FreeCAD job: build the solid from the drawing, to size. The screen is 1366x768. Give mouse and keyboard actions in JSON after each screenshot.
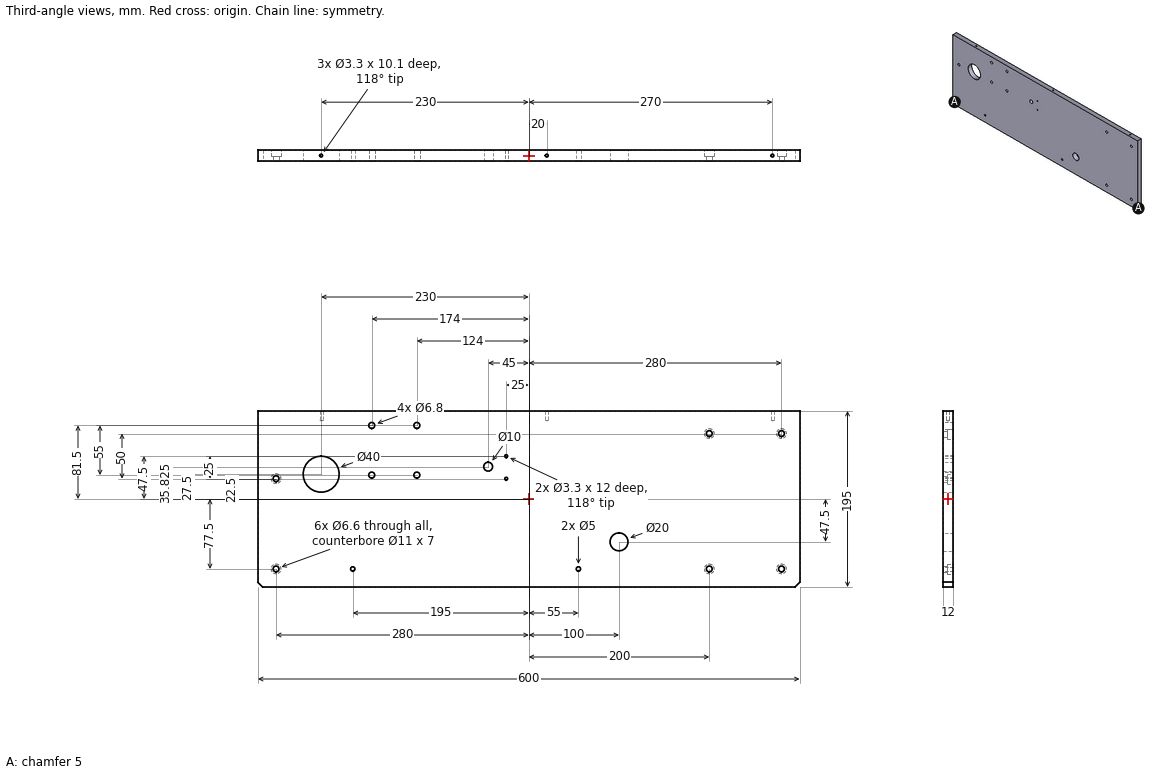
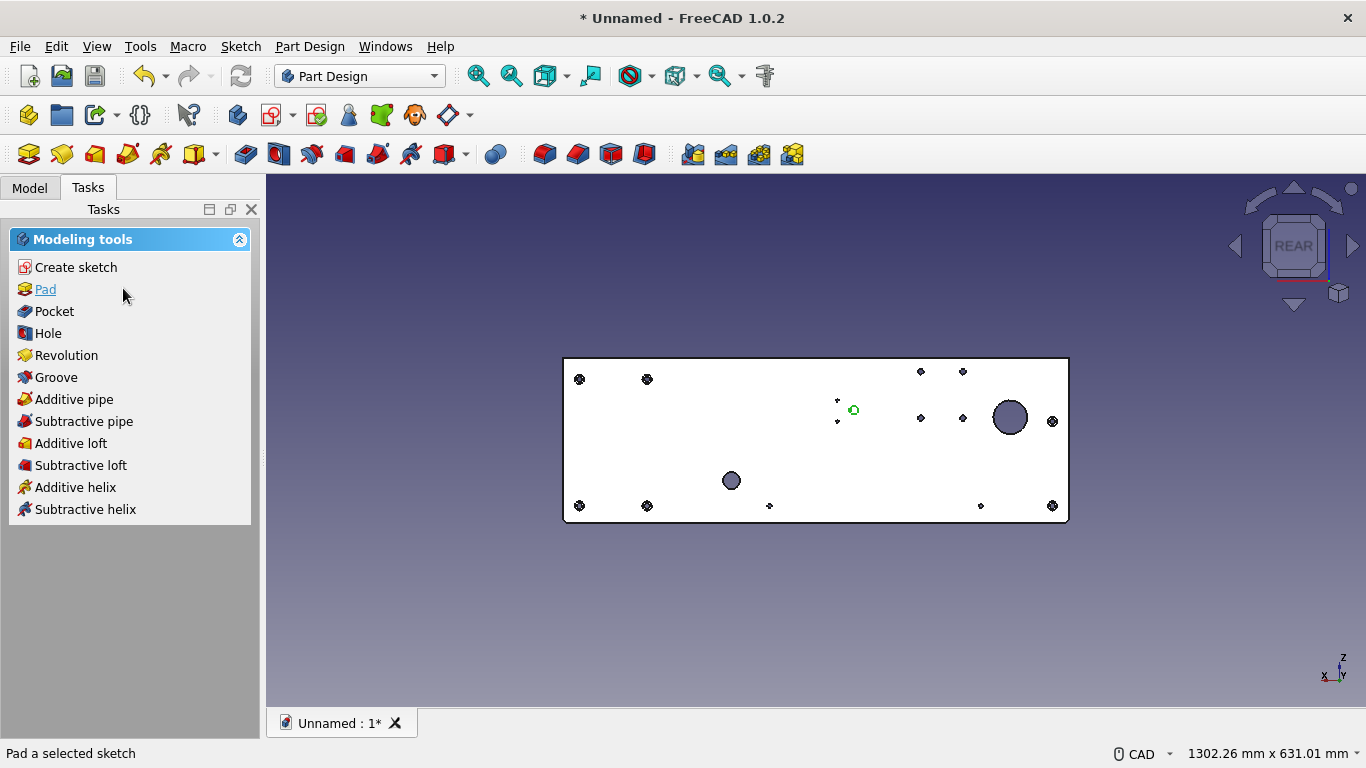
{"action": "left_click", "coordinate": [246, 154]}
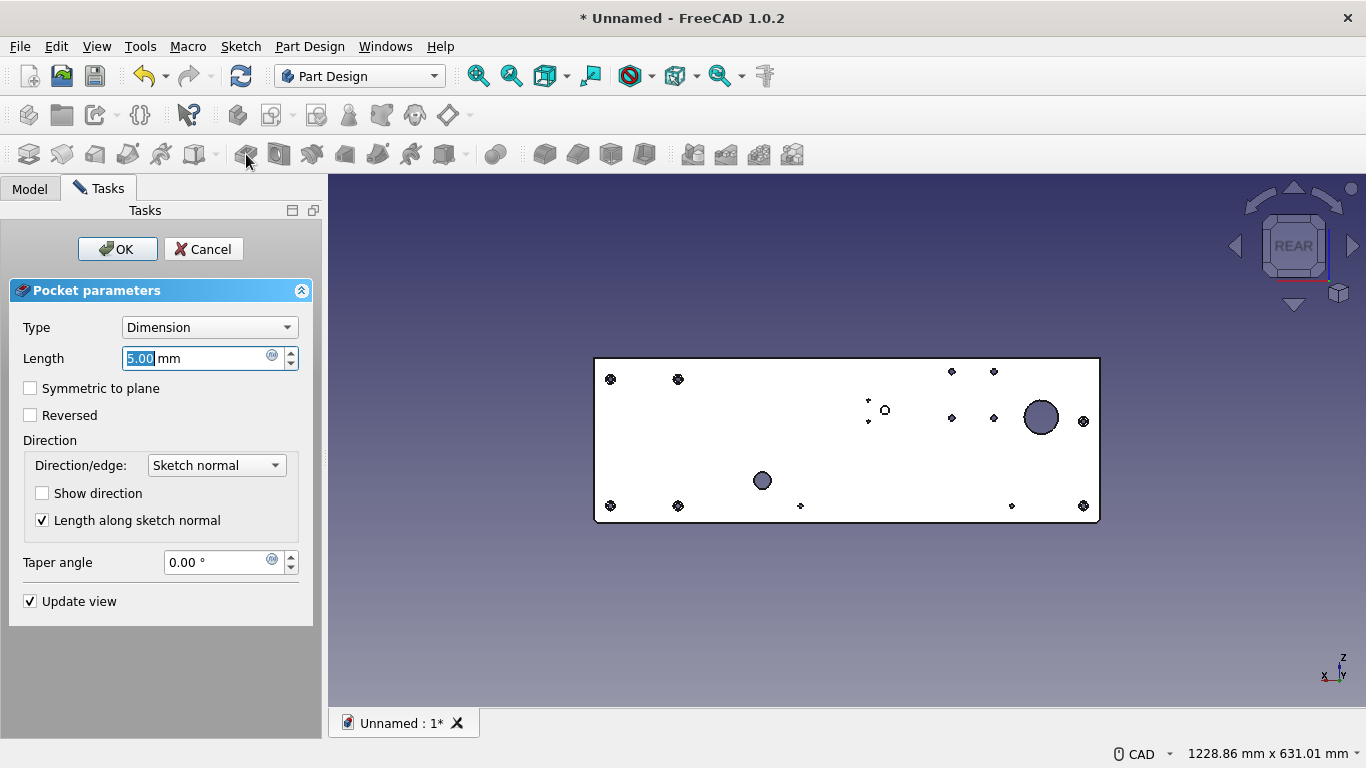
{"action": "left_click", "coordinate": [210, 328]}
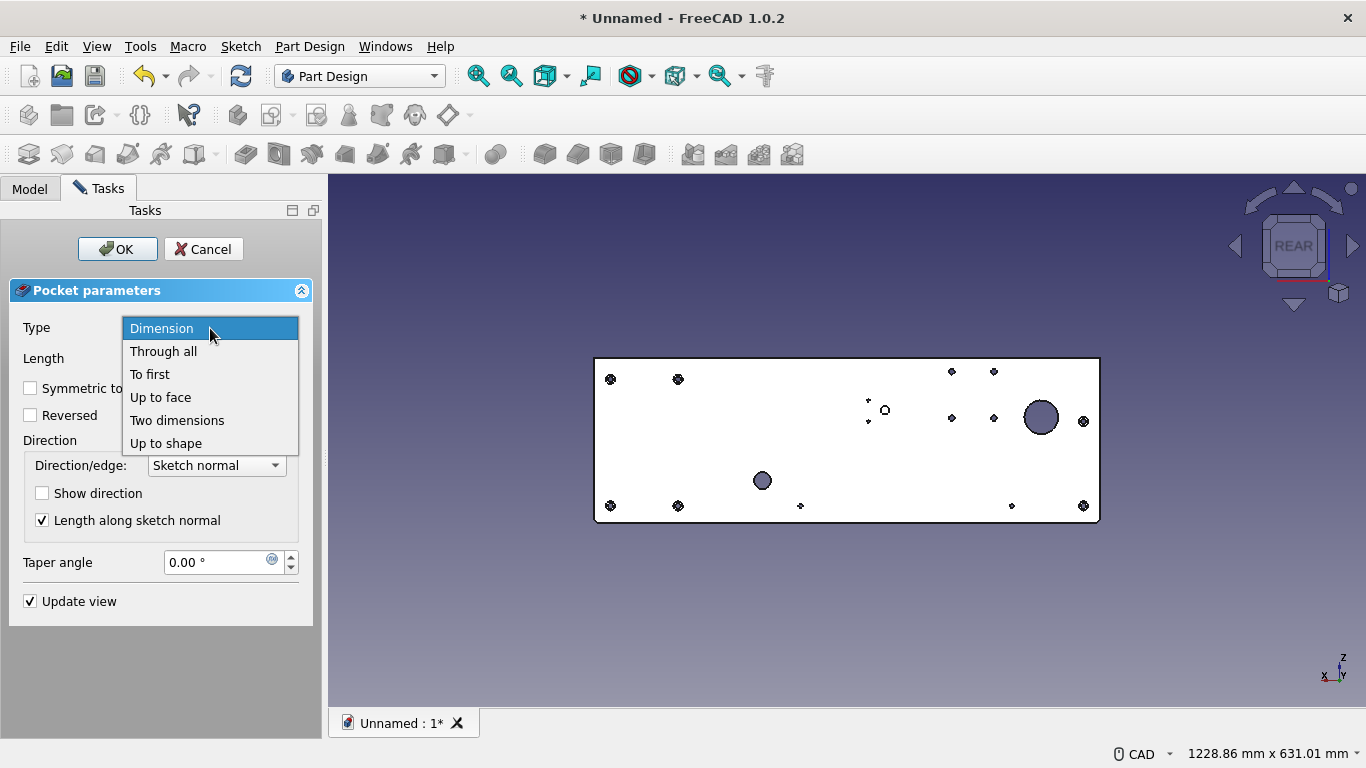
{"action": "left_click", "coordinate": [208, 352]}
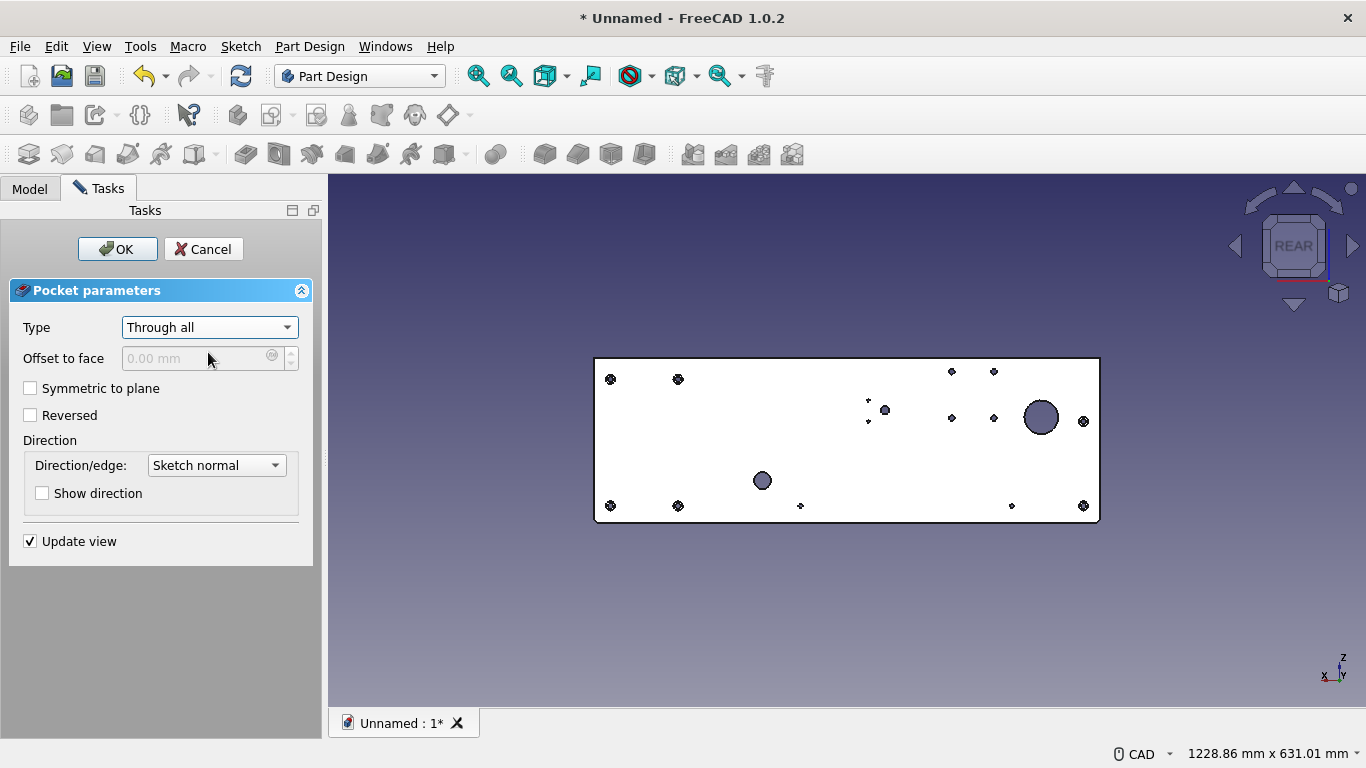
{"action": "left_click", "coordinate": [118, 249]}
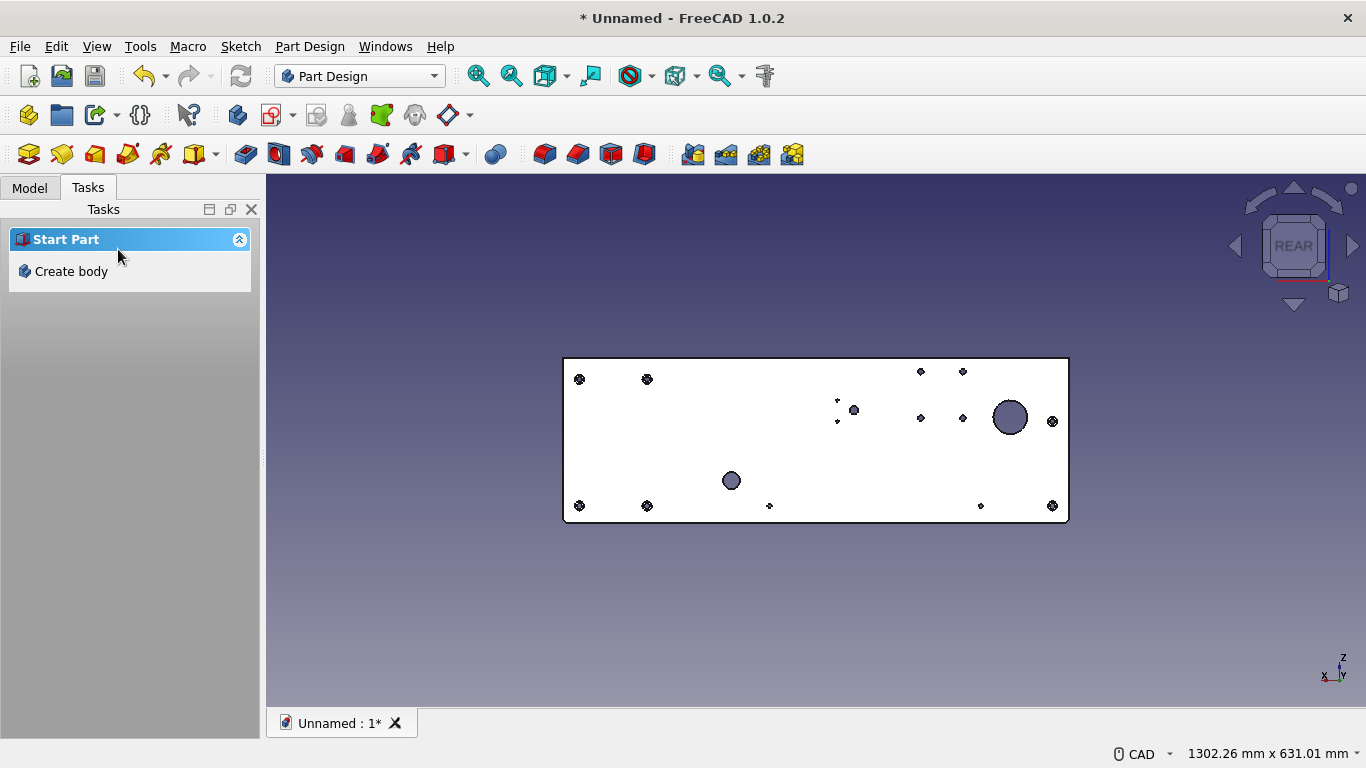
{"action": "key", "text": "0"}